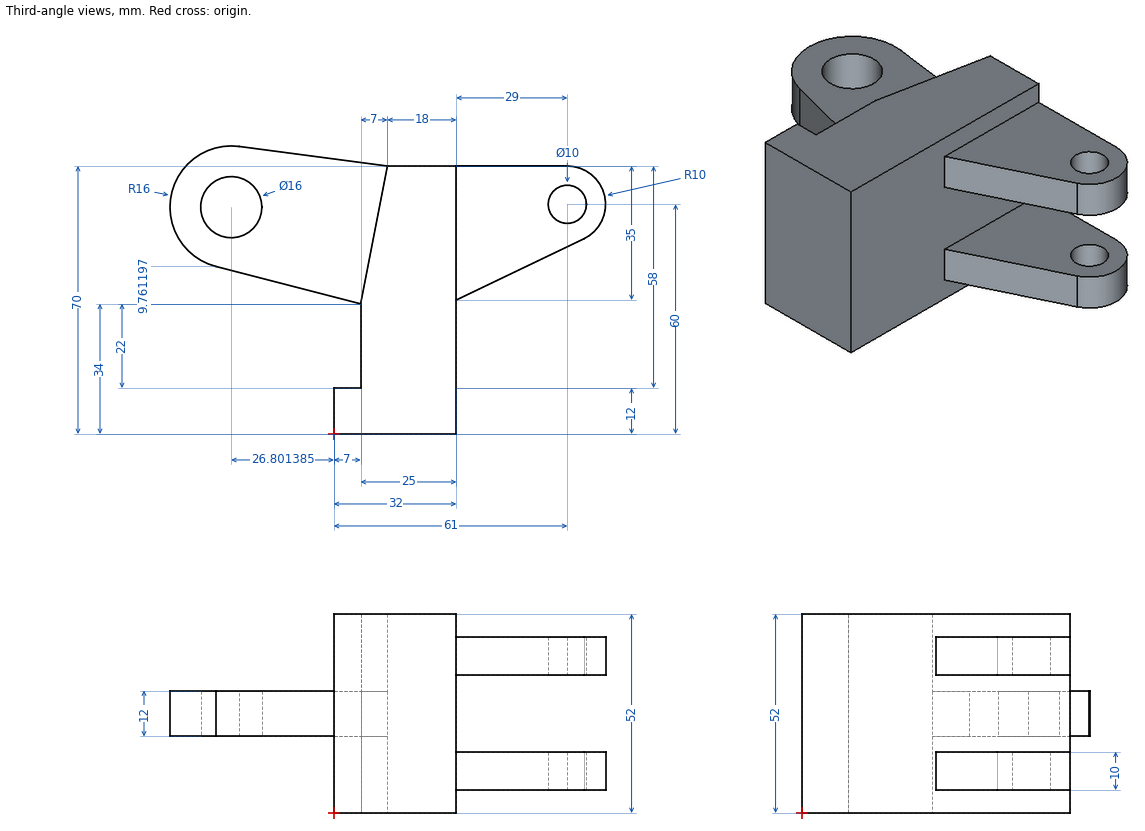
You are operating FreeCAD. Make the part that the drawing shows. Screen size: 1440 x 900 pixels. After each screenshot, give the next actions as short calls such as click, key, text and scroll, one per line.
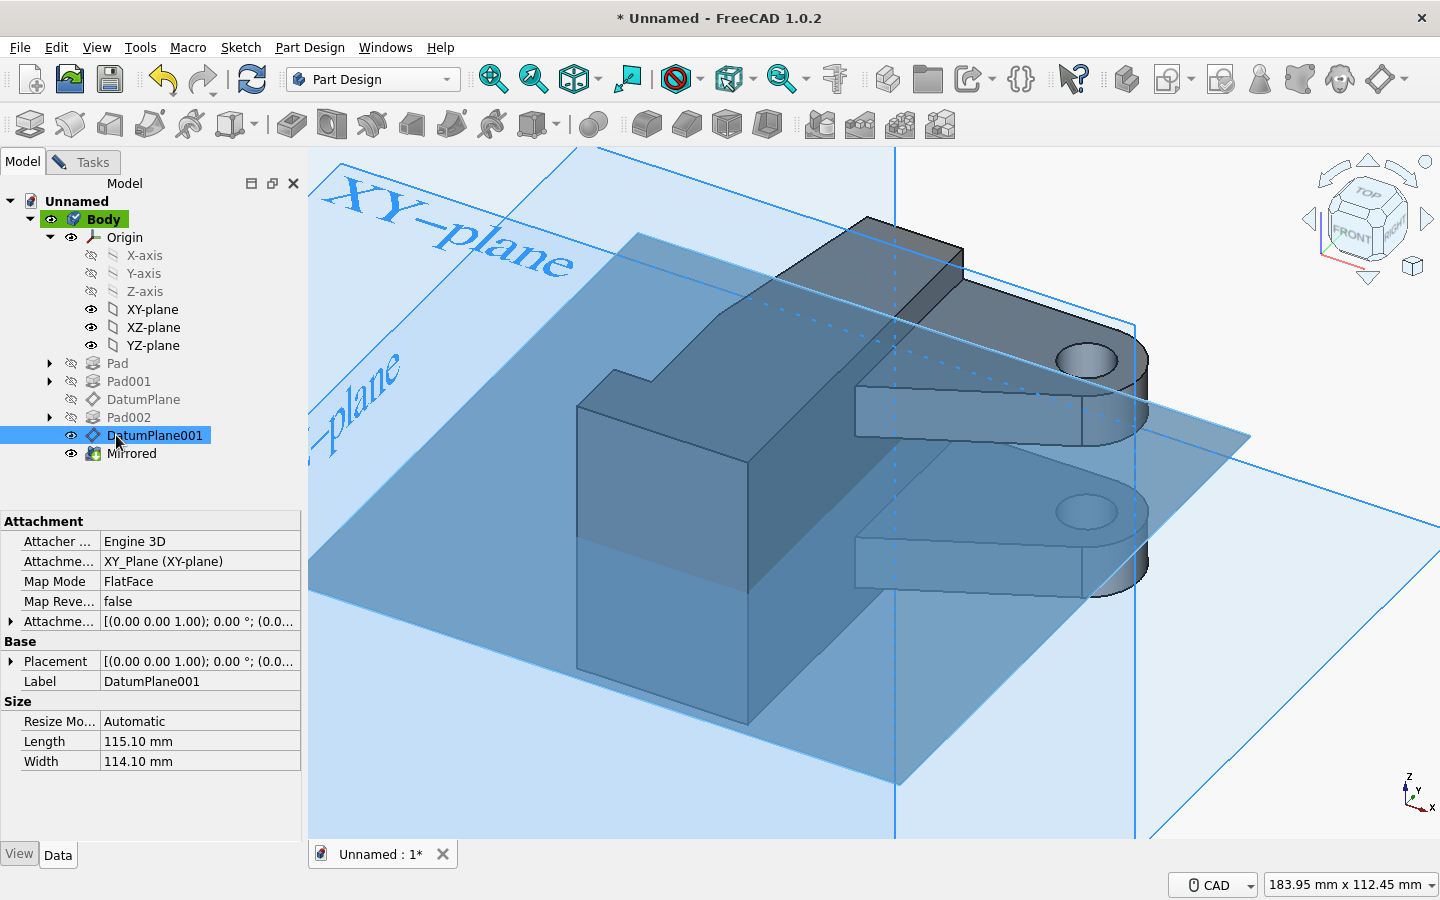
click(84, 161)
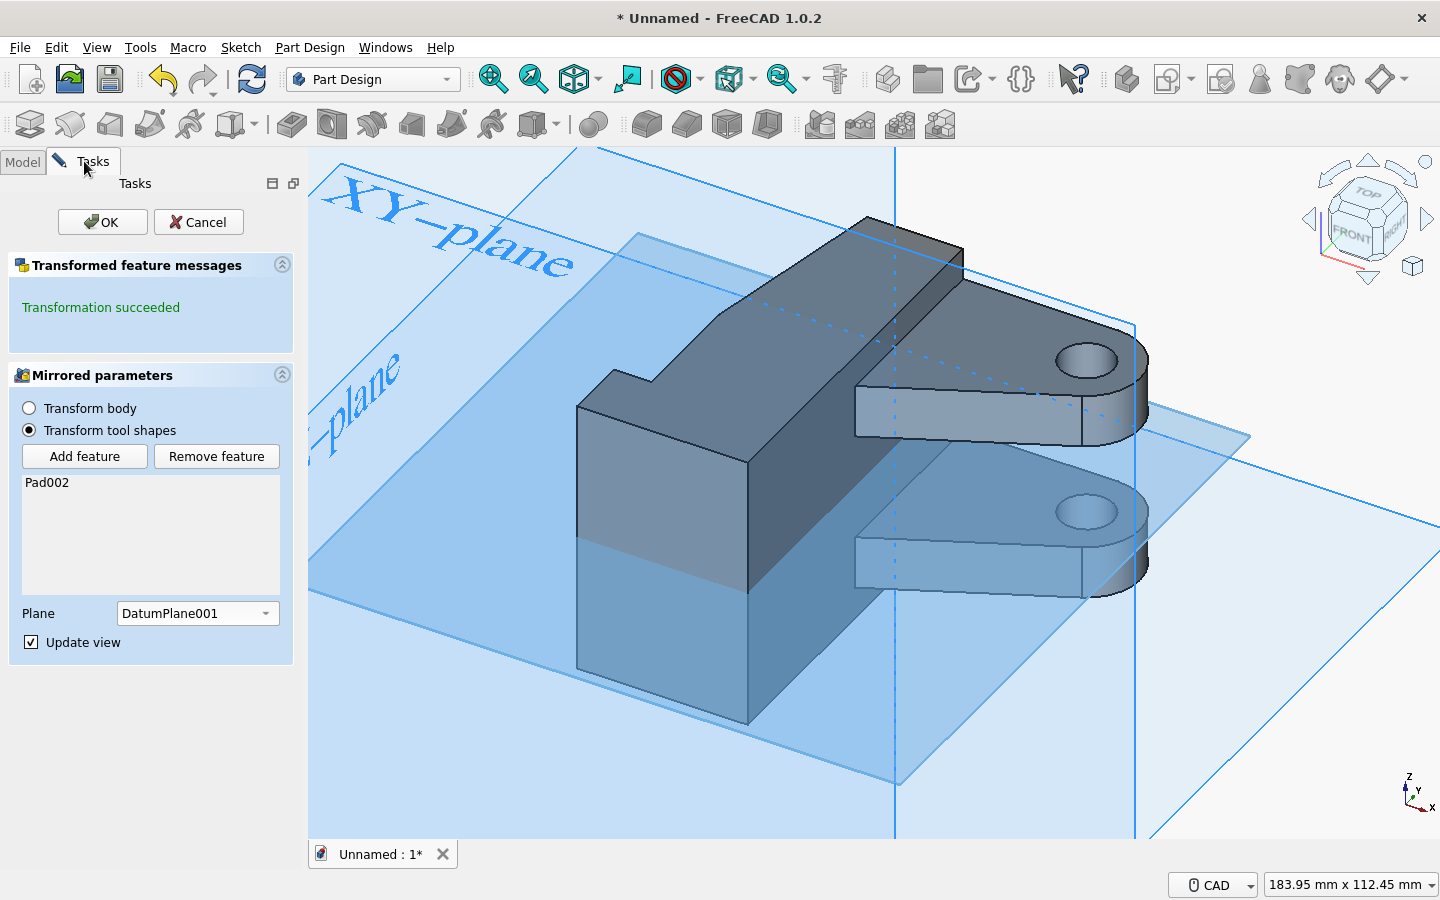
click(103, 222)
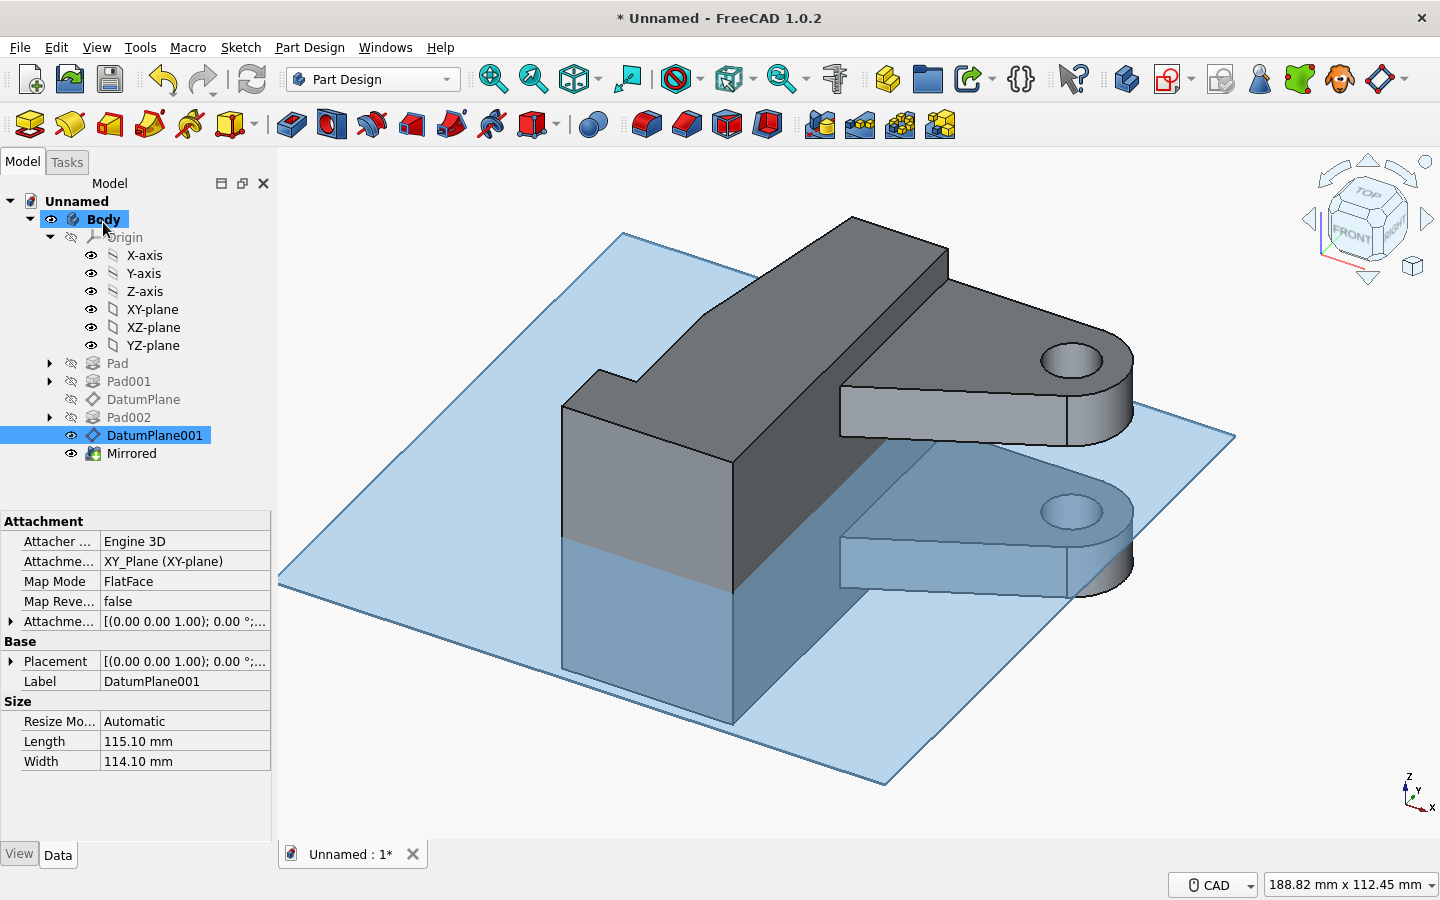
click(116, 435)
key(space)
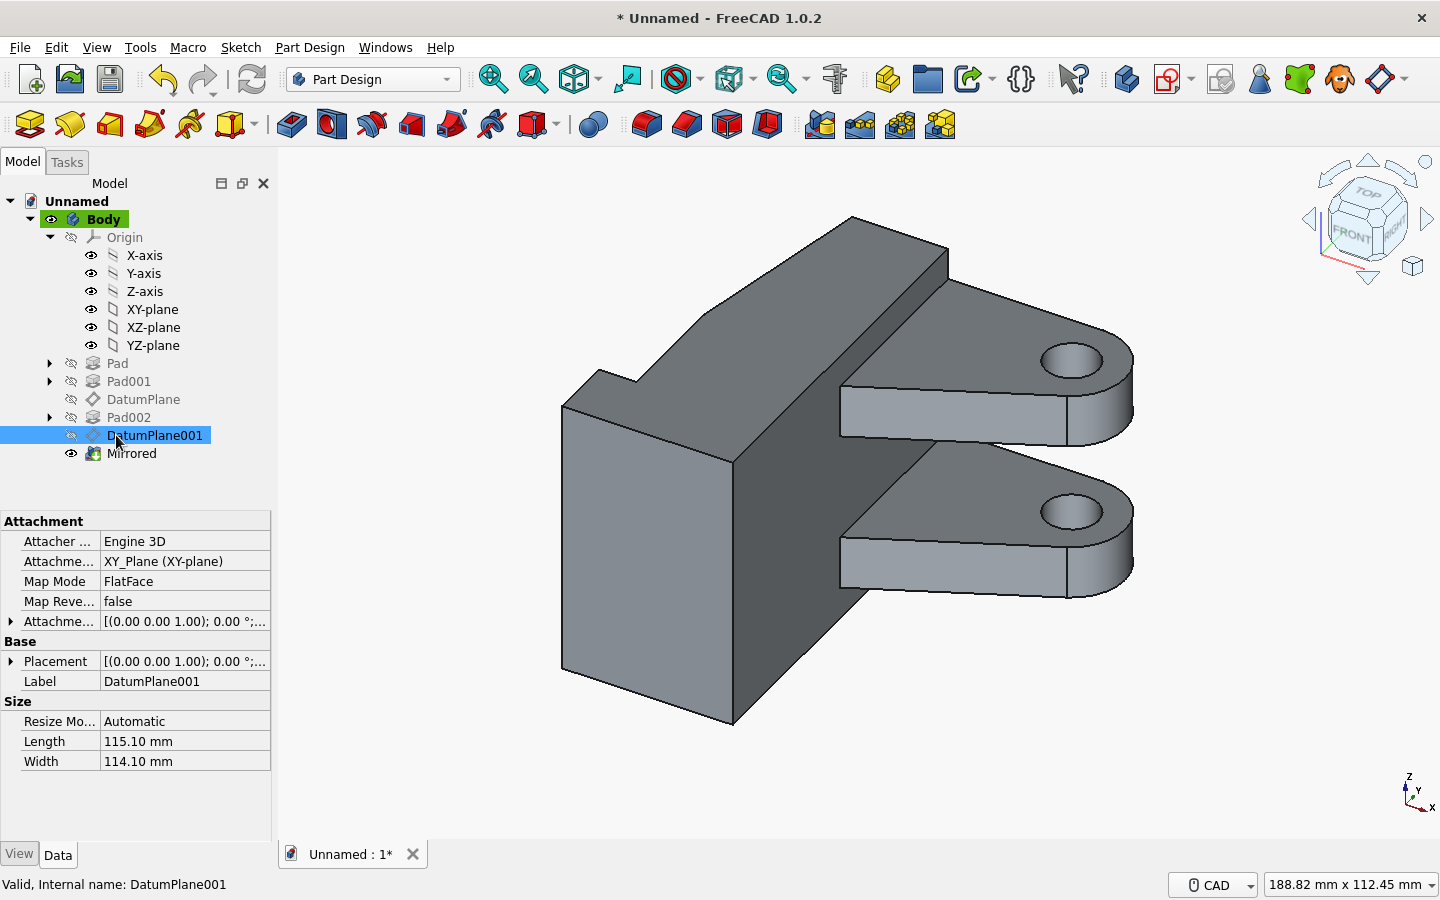
click(136, 309)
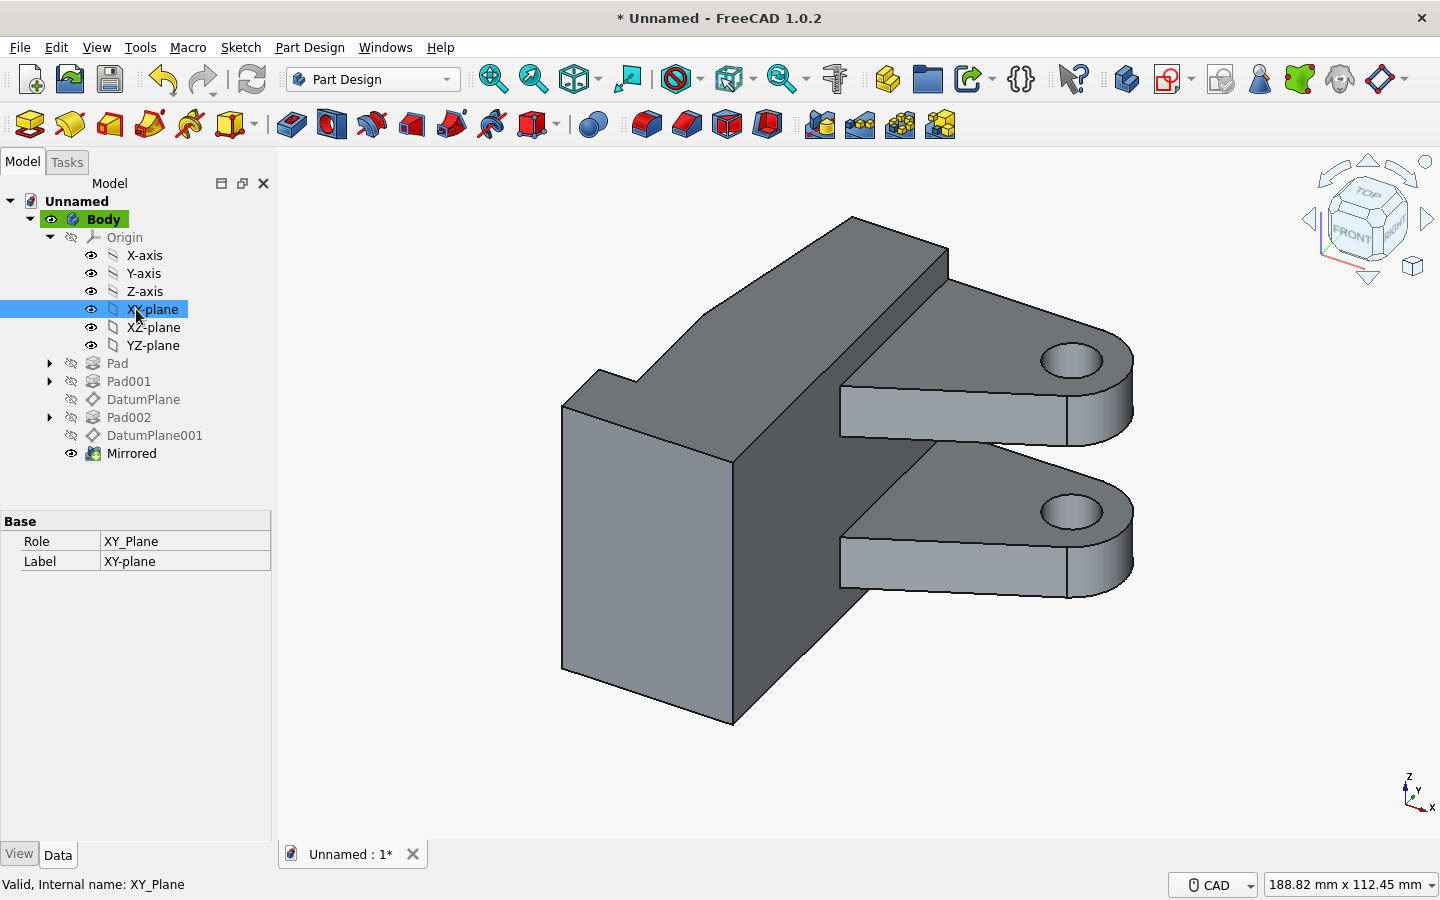
click(1380, 80)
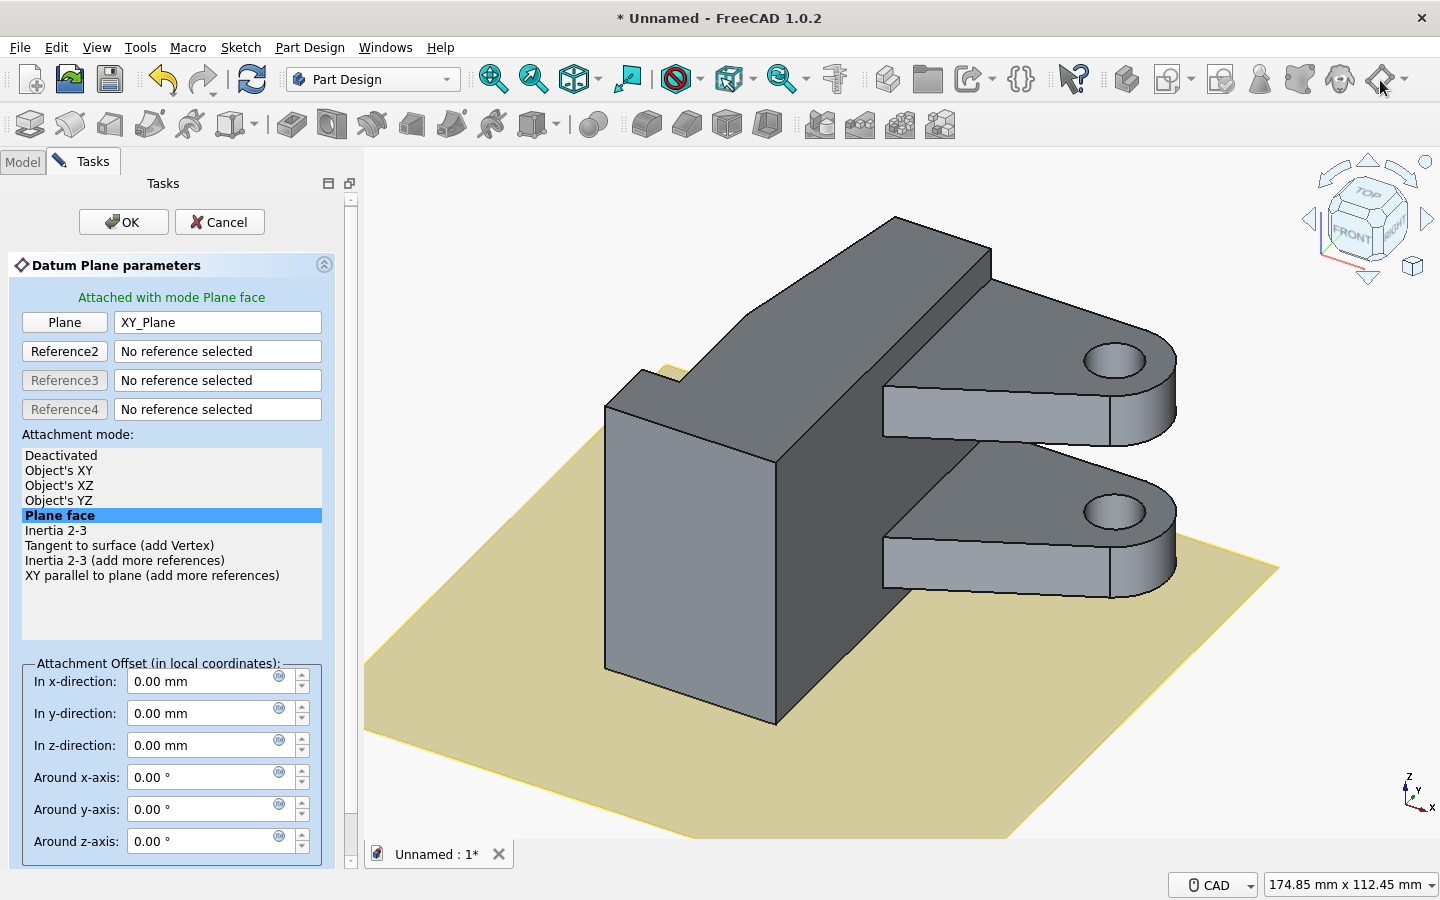
triple_click(210, 745)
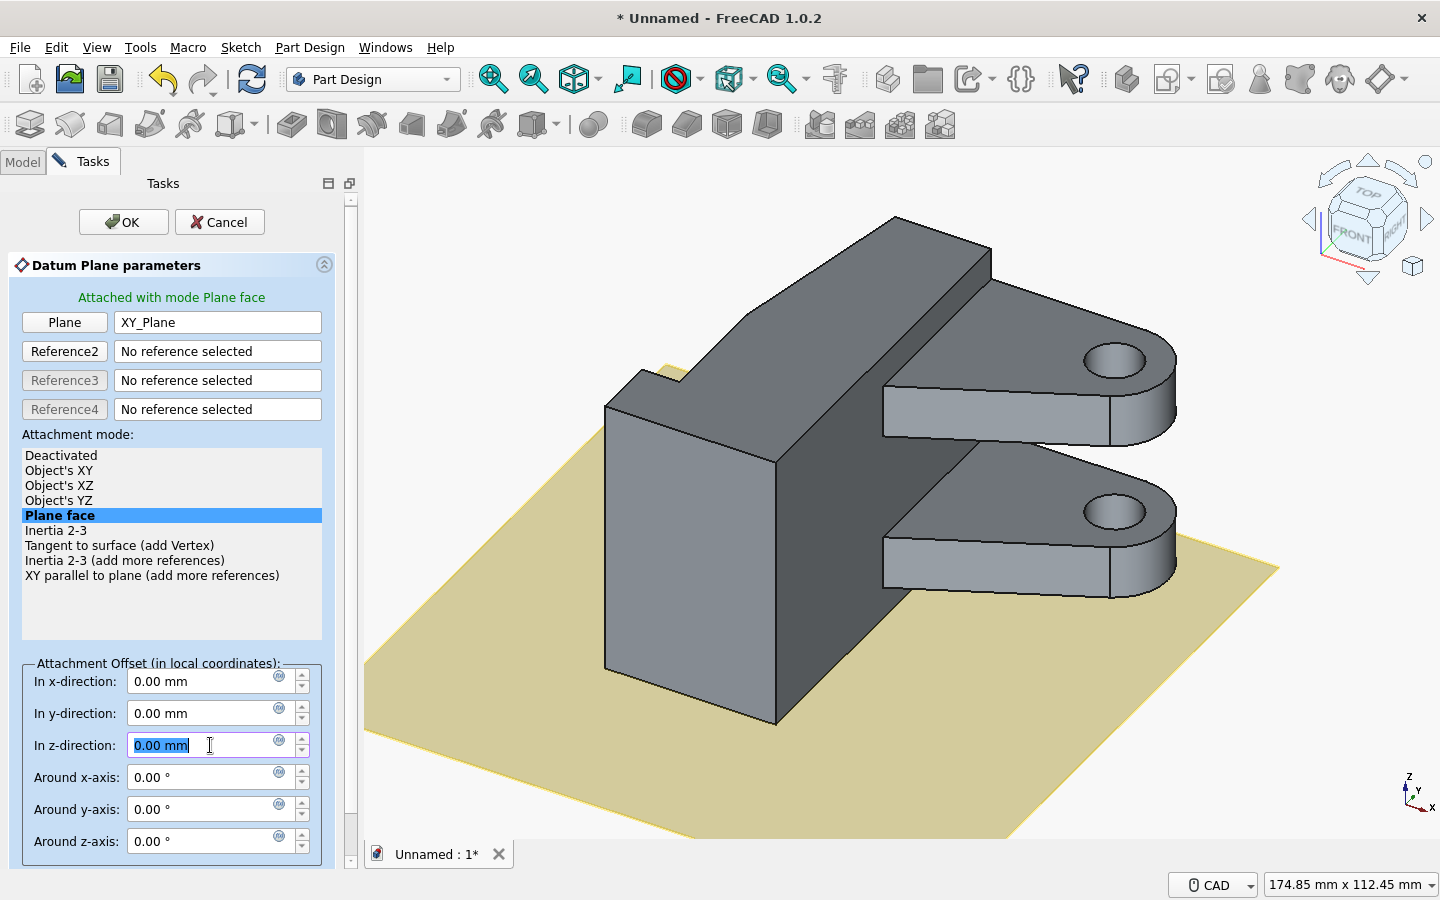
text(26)
key(Tab)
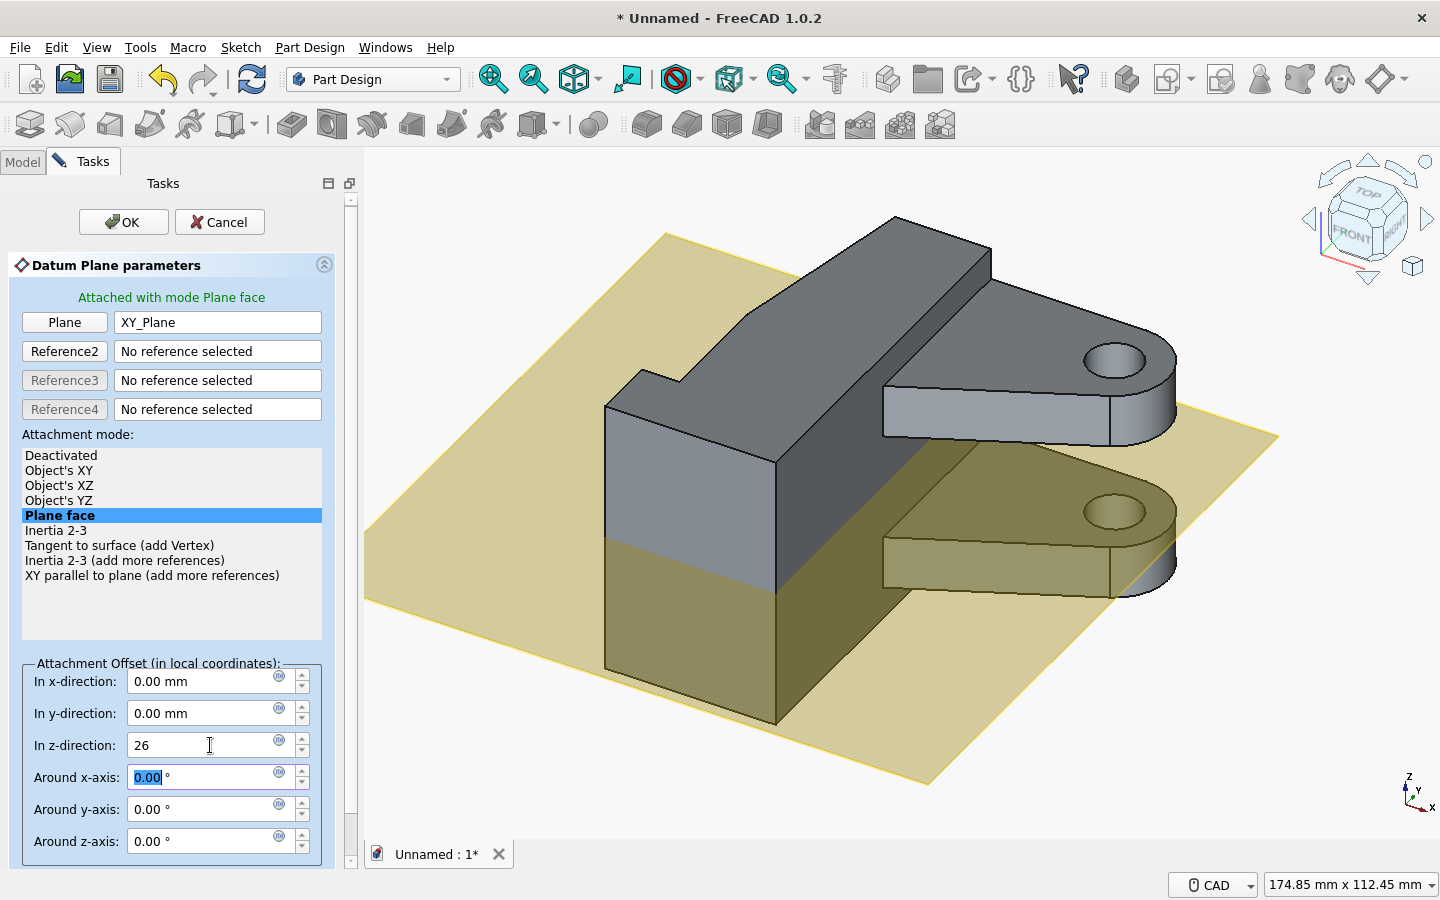
click(124, 222)